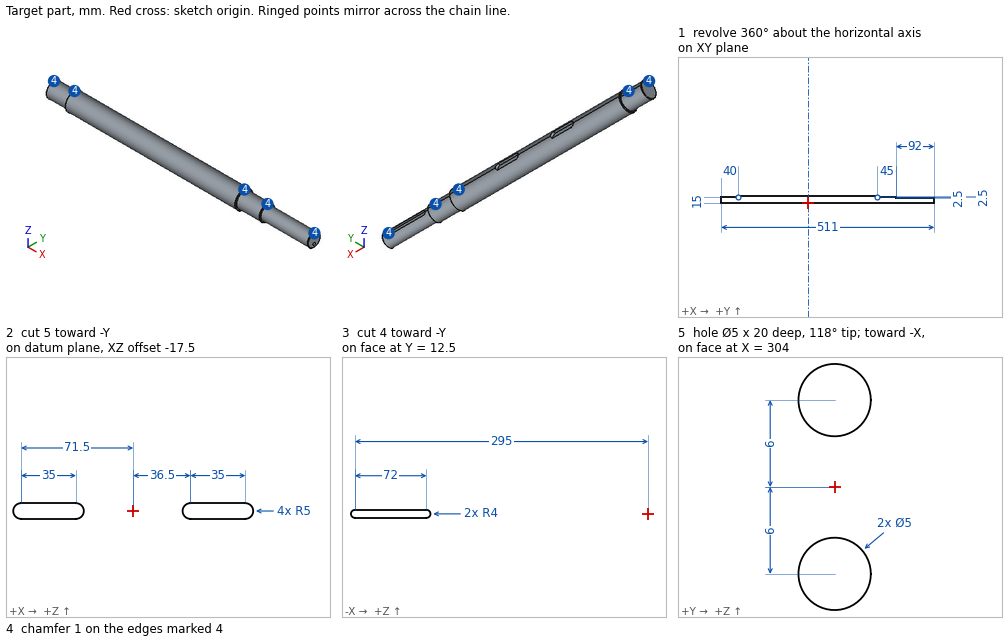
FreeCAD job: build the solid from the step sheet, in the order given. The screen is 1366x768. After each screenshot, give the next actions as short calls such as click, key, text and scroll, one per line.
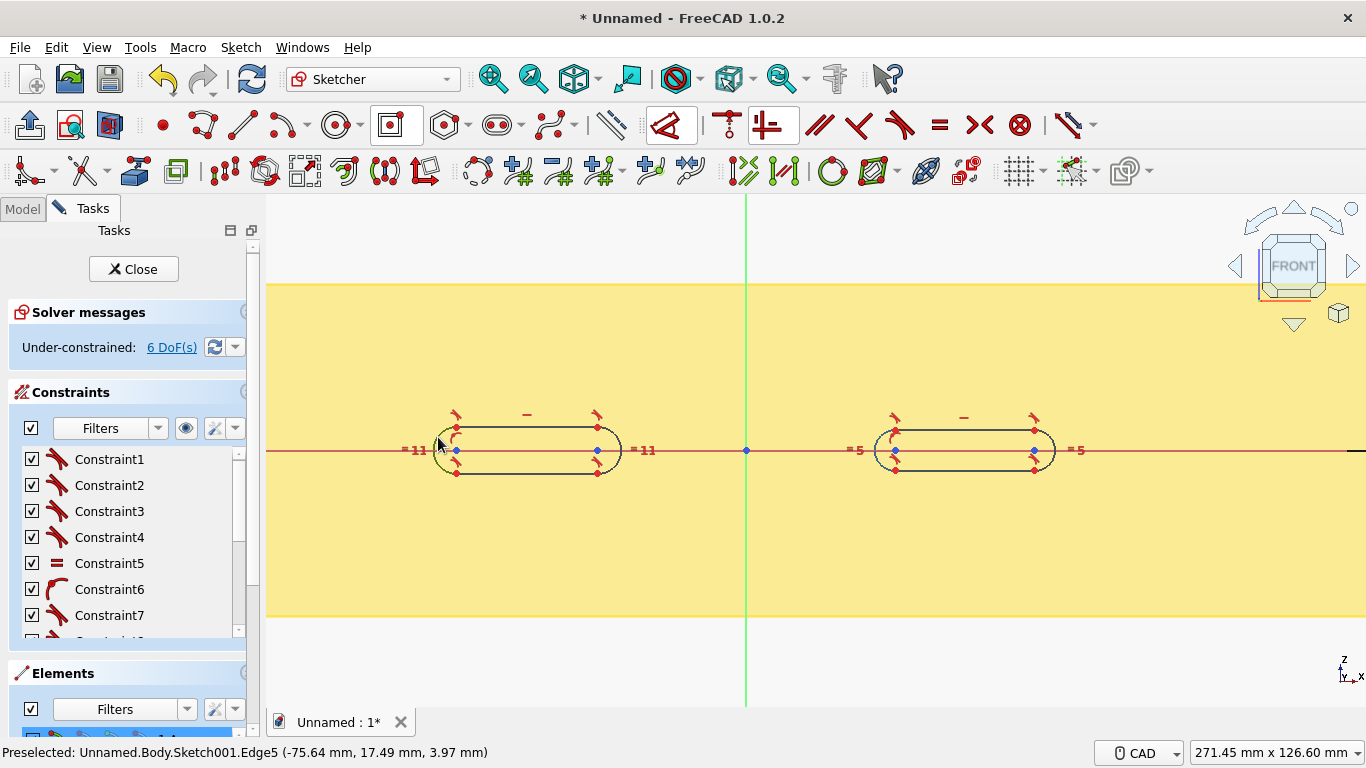
click(940, 126)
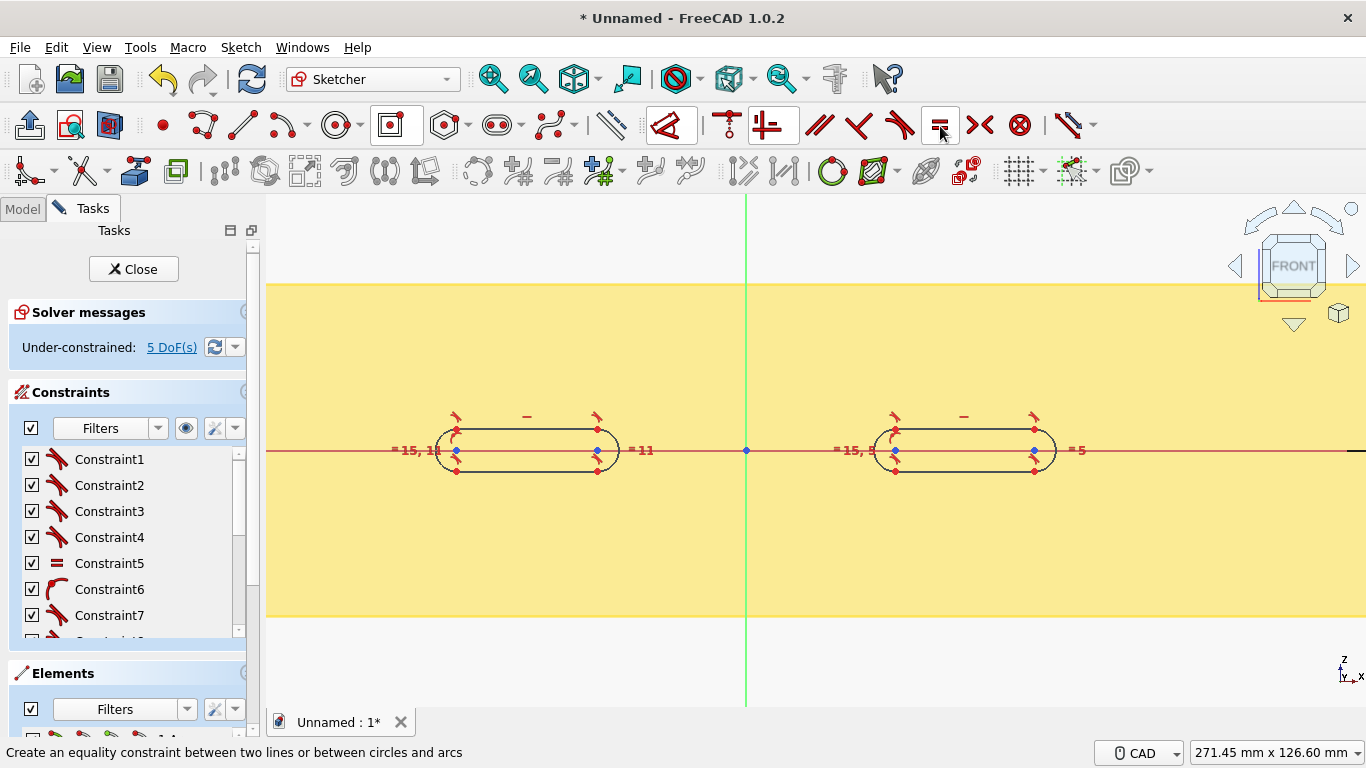
scroll(878, 438, up, 4)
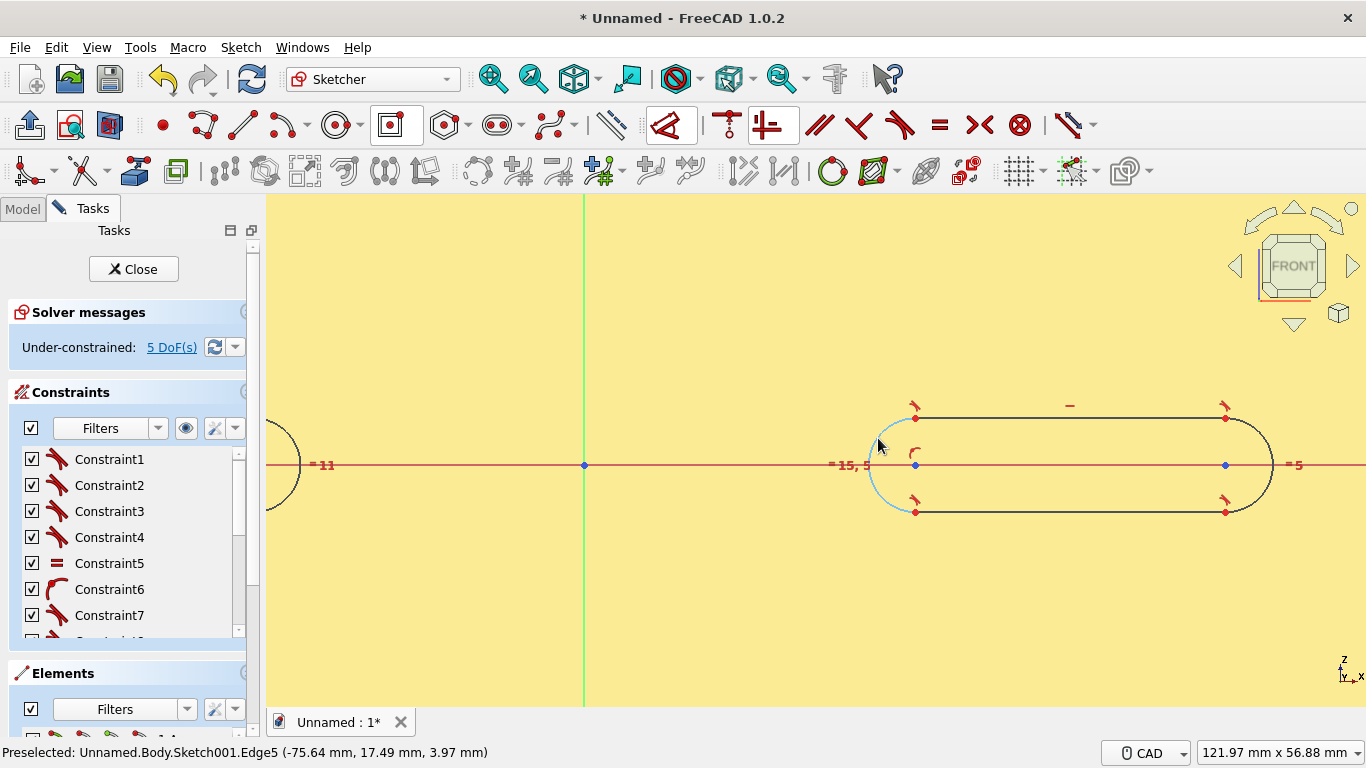
click(878, 438)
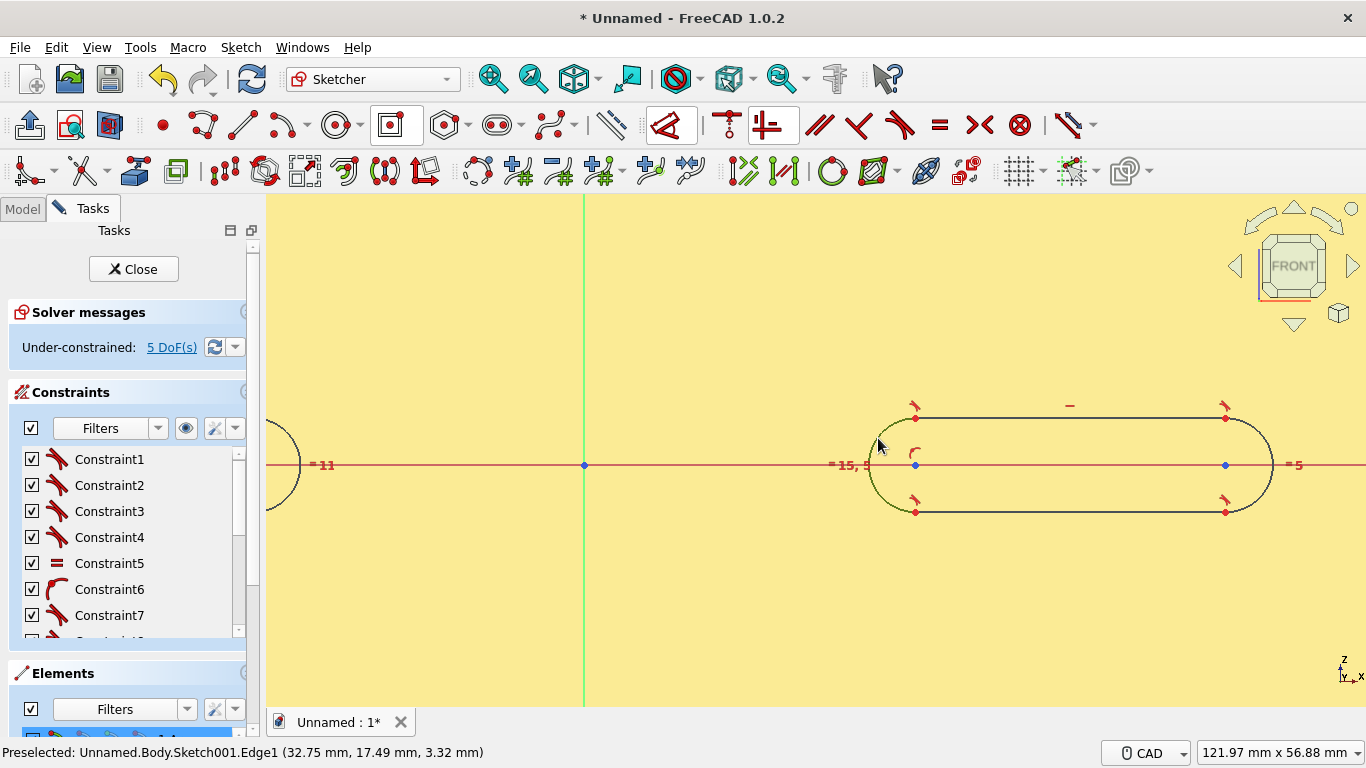
key(k)
key(r)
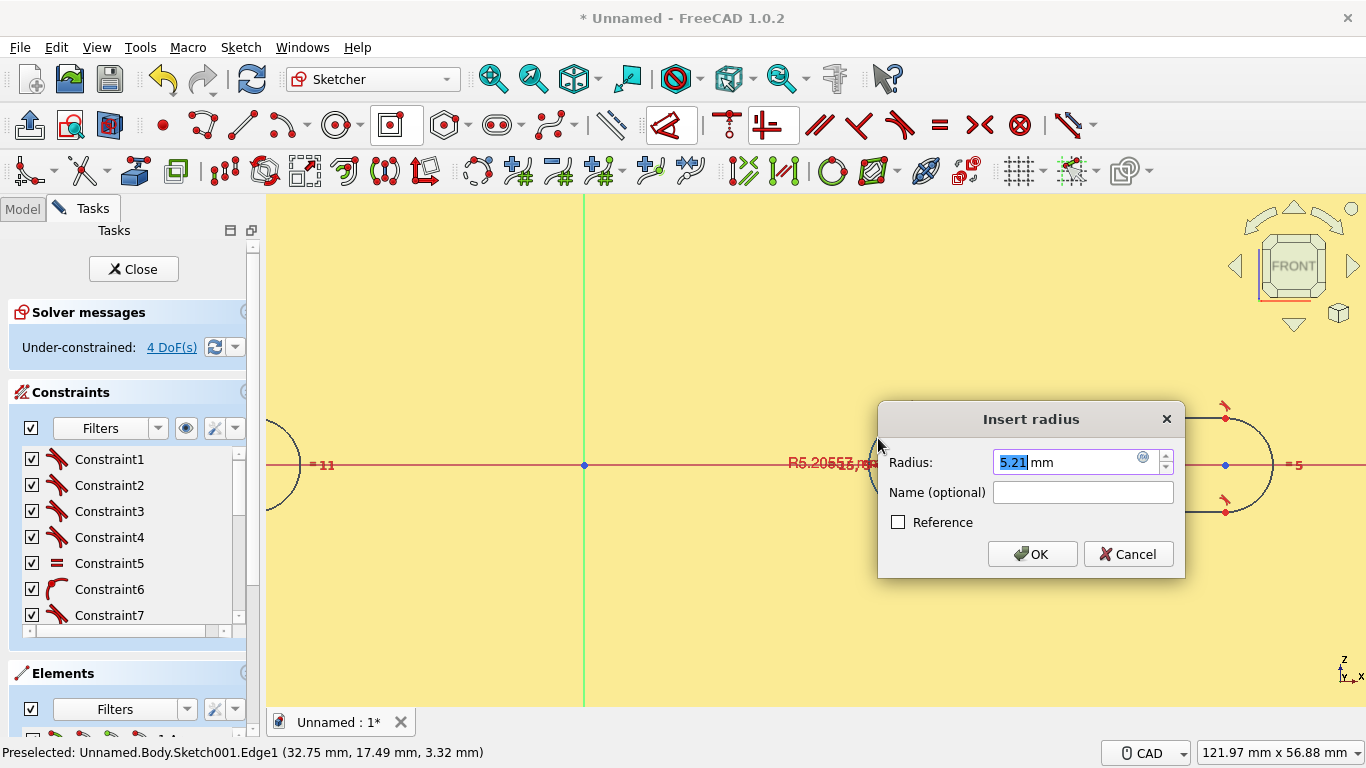
text(5)
key(Return)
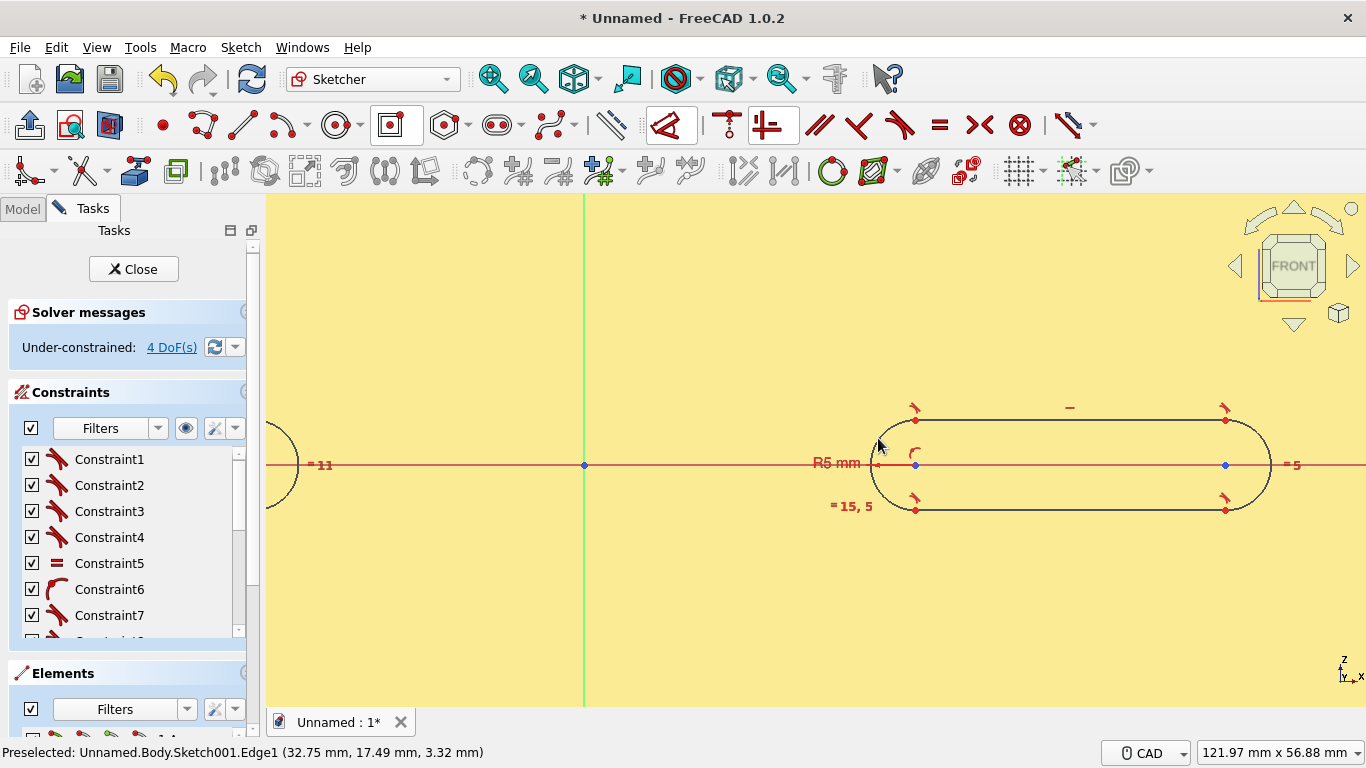
click(1009, 420)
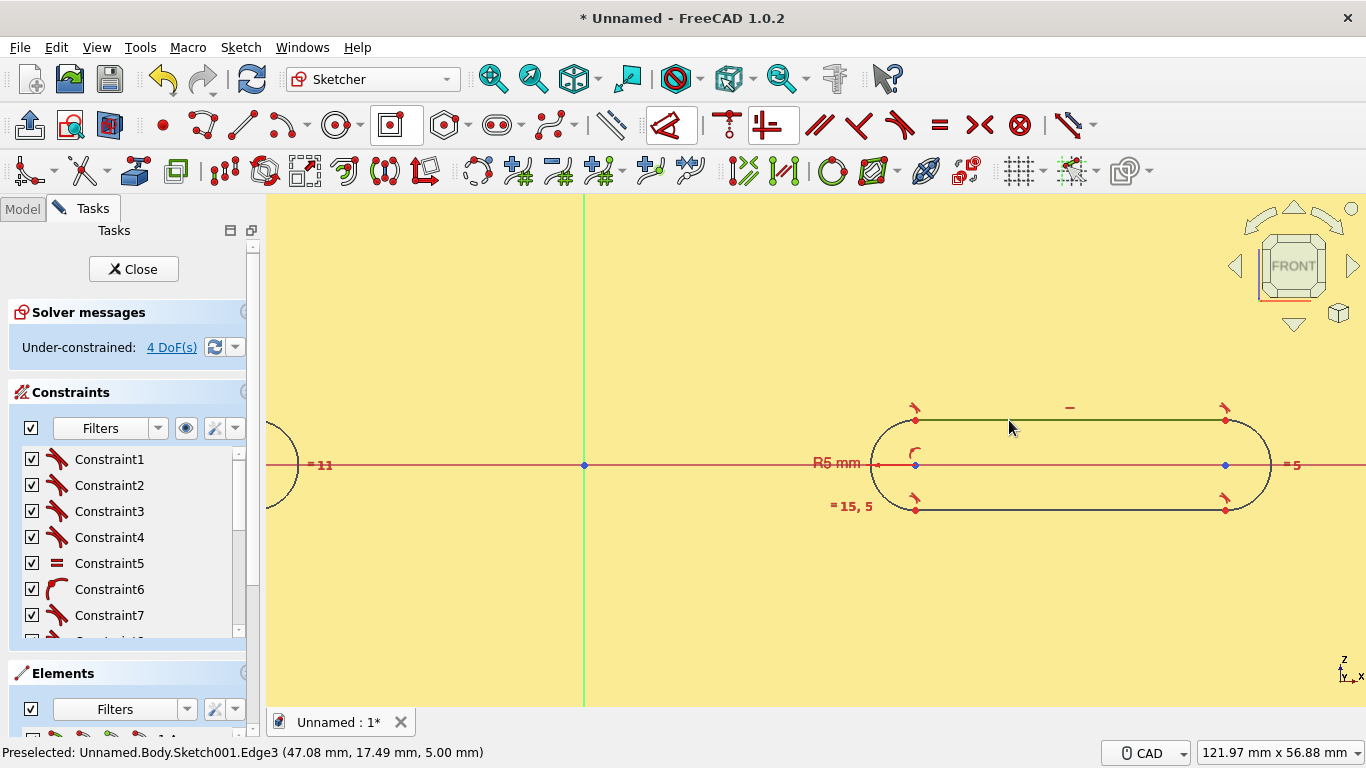
key(l)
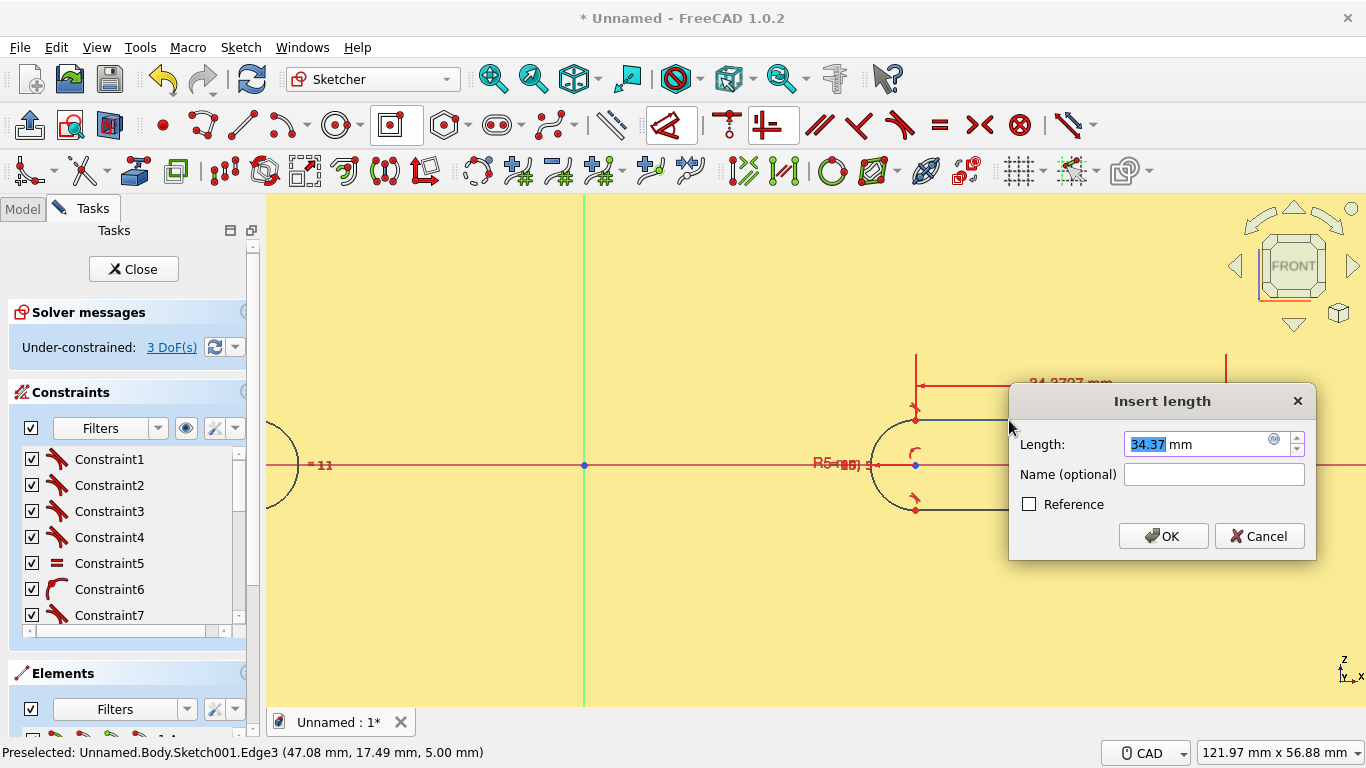
text(35)
key(Return)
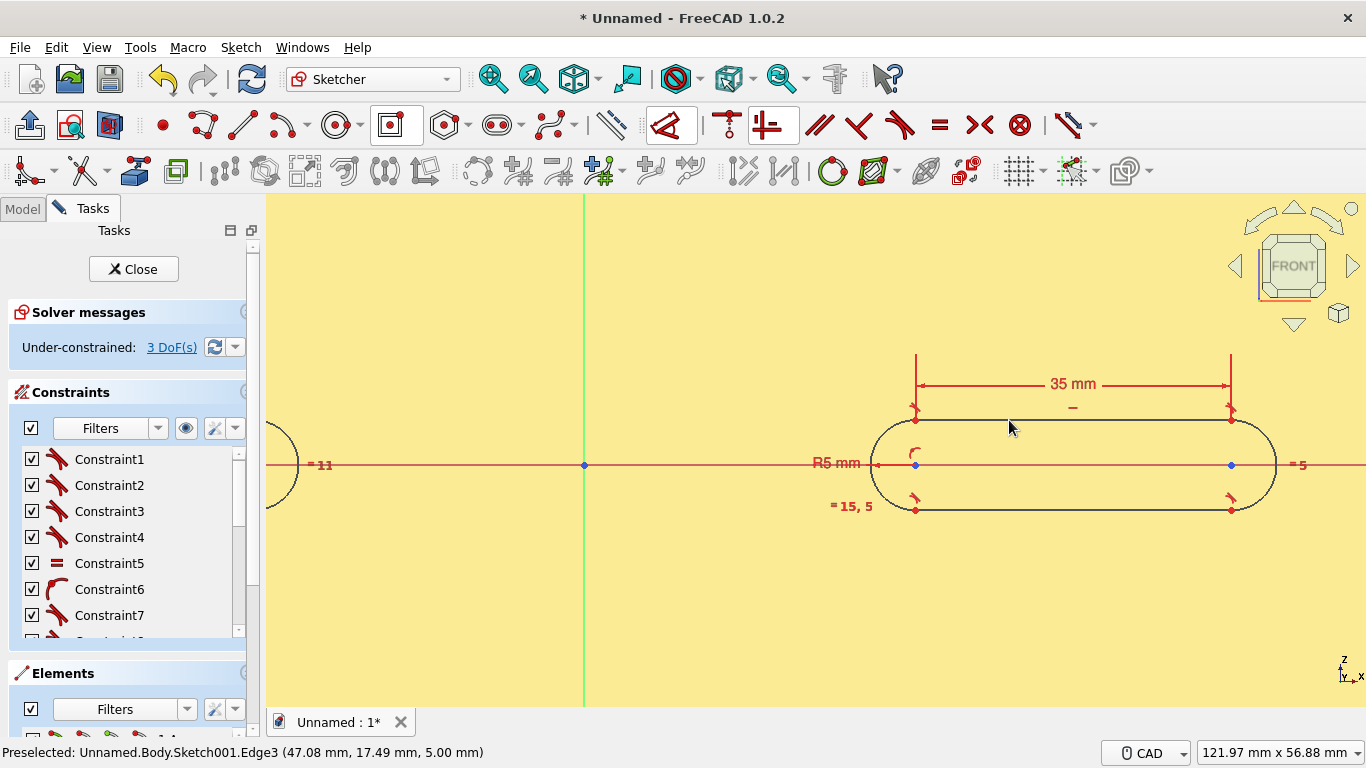
scroll(881, 438, down, 4)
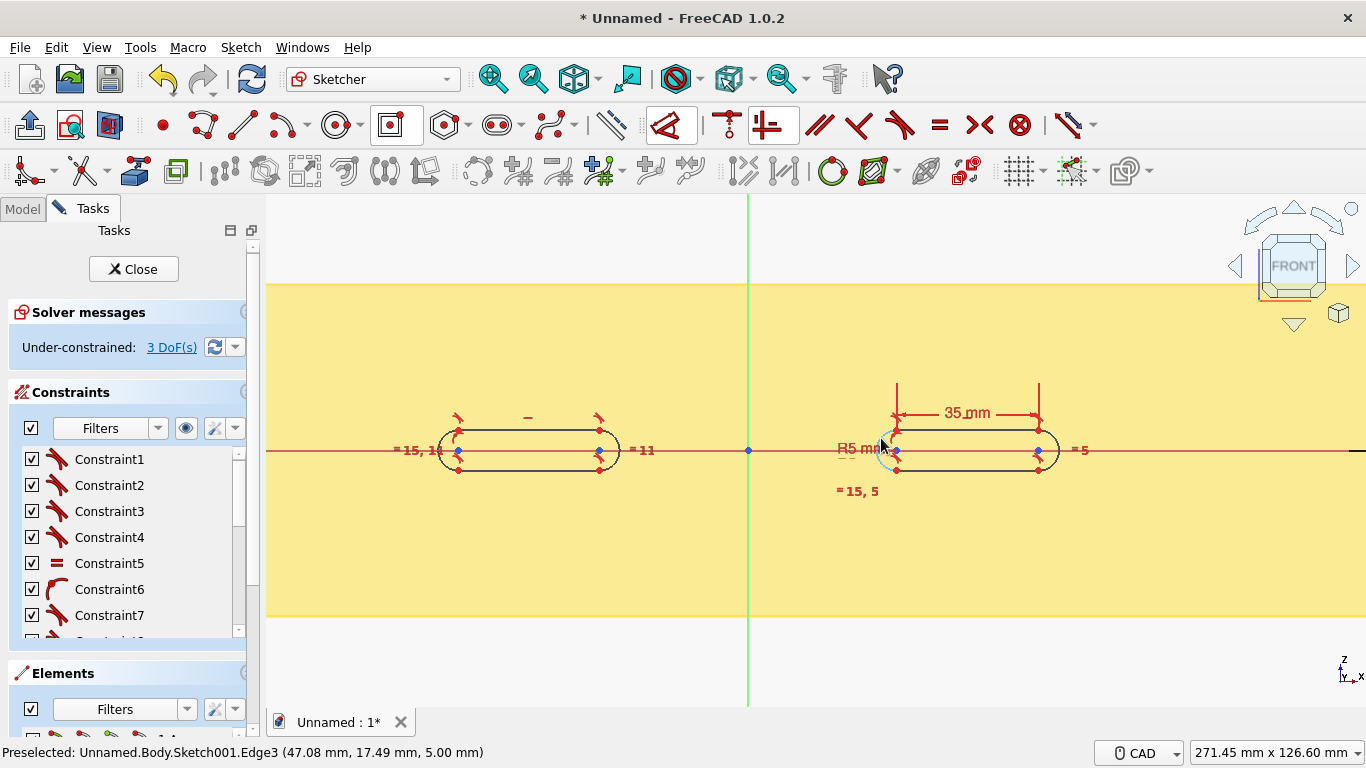
click(501, 430)